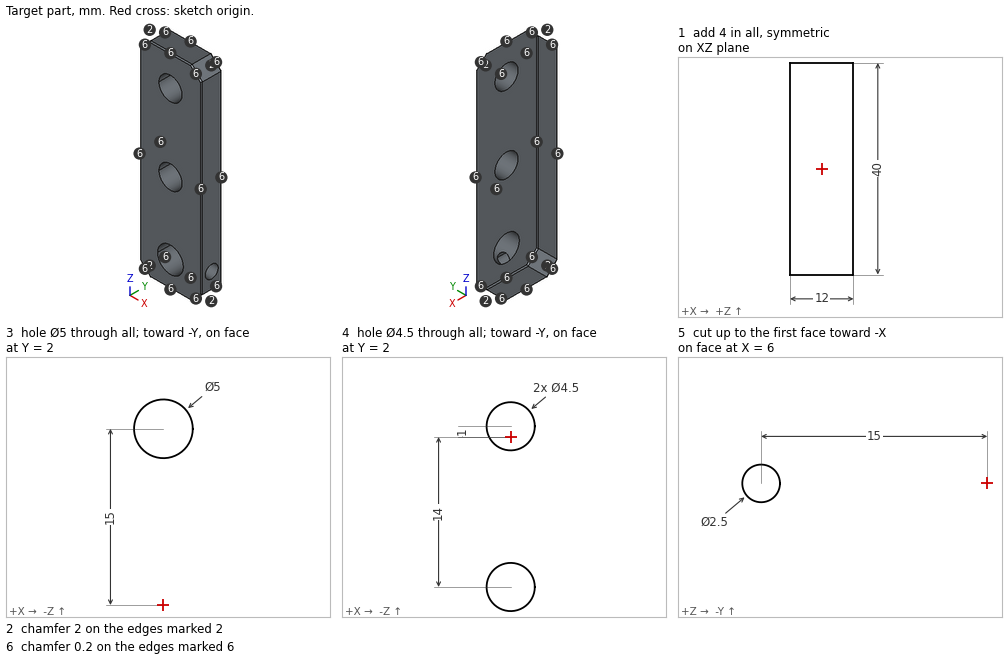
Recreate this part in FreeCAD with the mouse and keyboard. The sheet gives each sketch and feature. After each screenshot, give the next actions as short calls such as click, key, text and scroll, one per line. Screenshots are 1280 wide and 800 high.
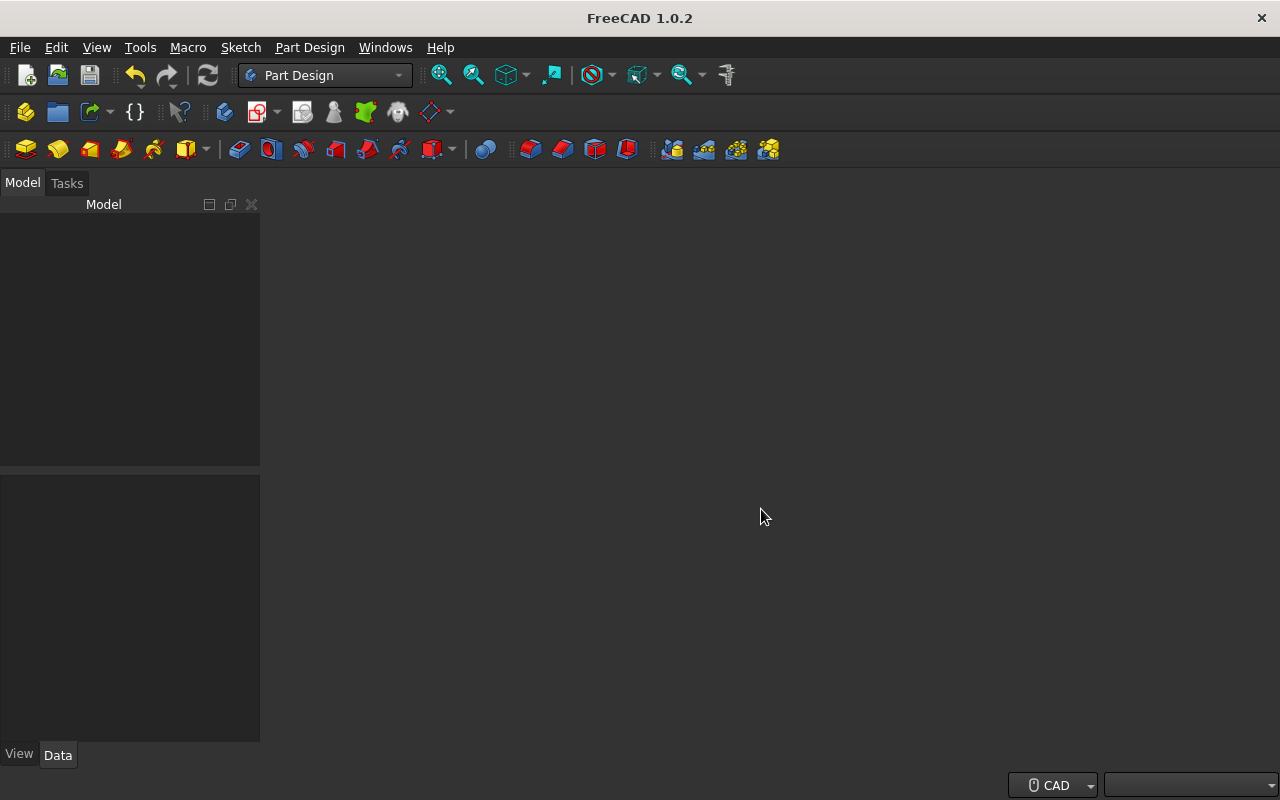
click(26, 76)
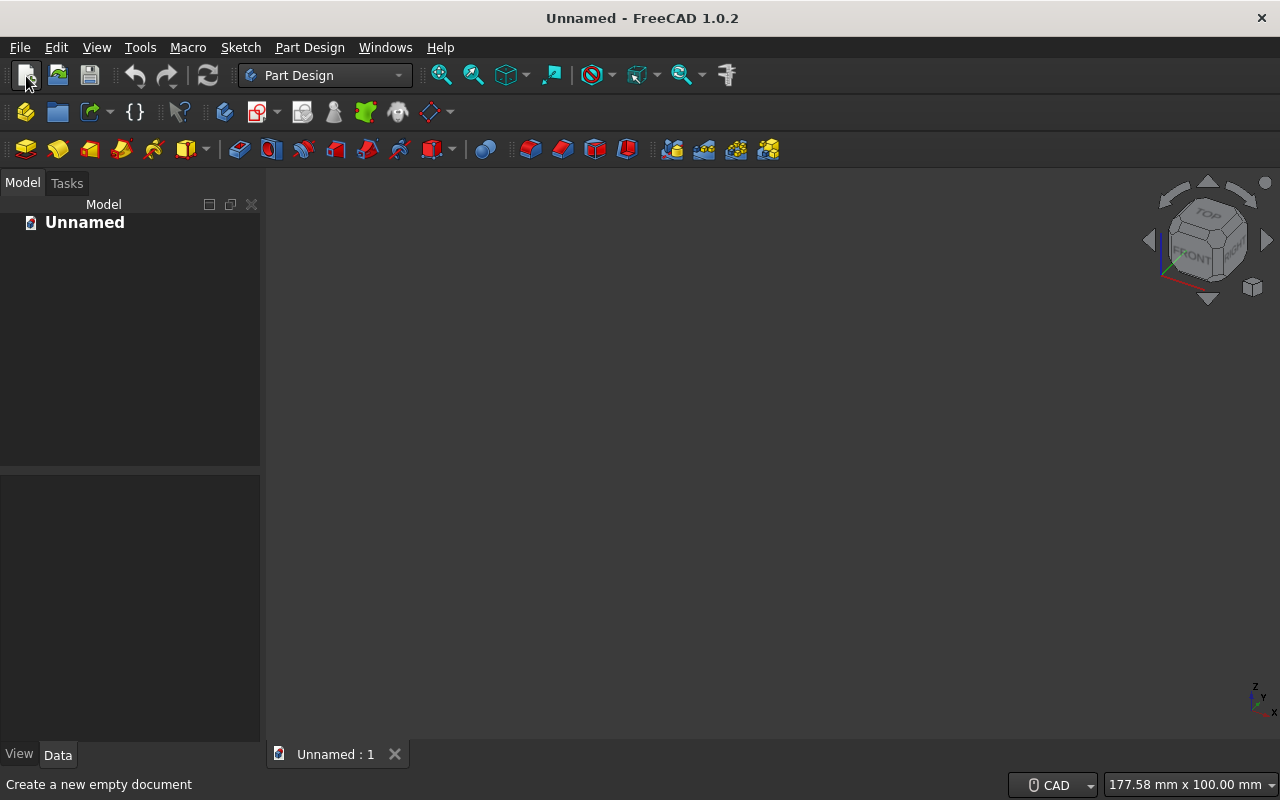
click(258, 112)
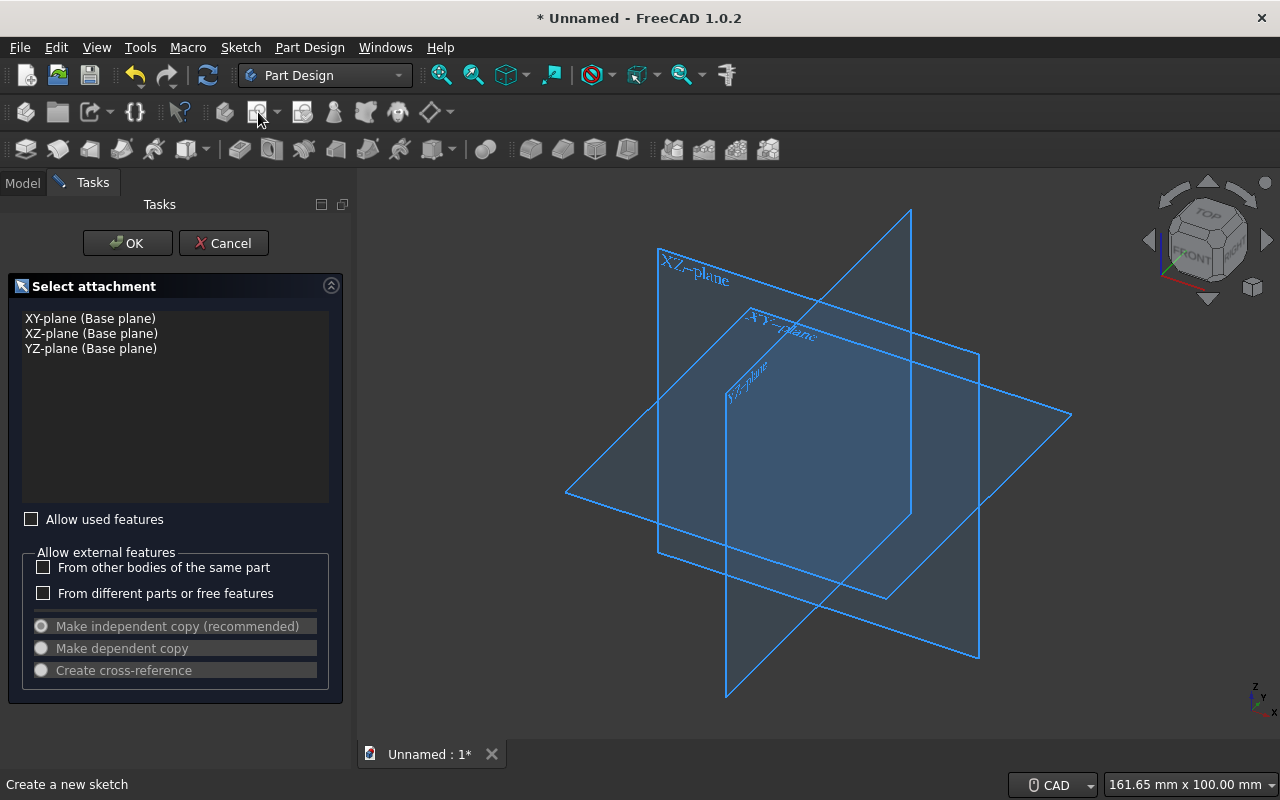
click(82, 334)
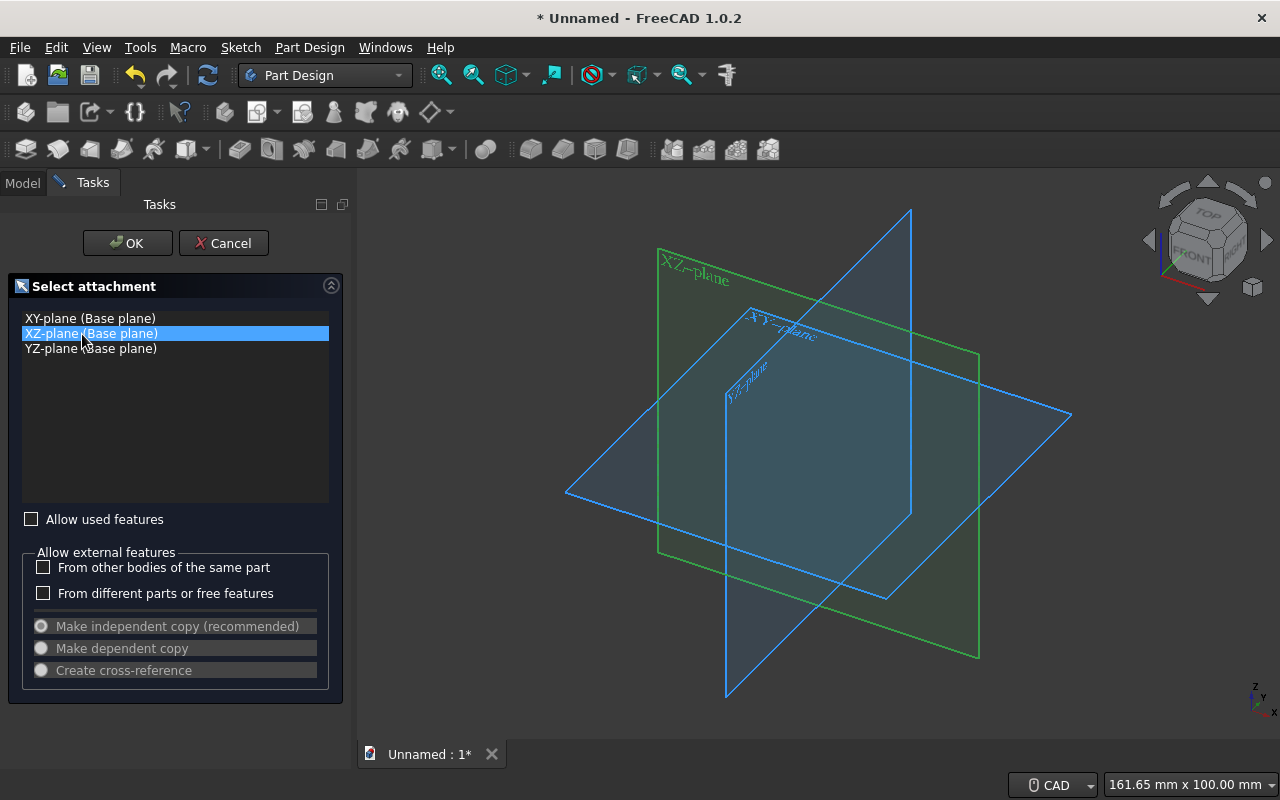
click(128, 243)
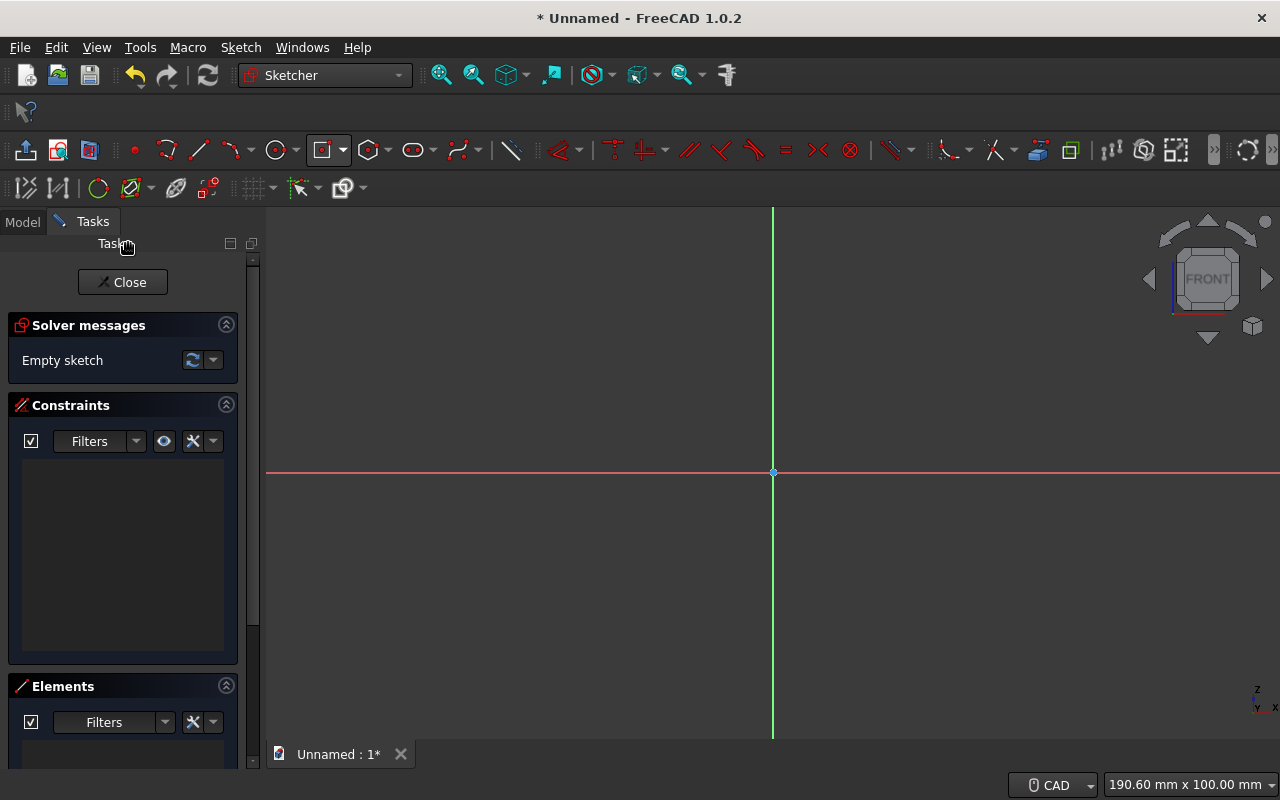
scroll(912, 473, up, 2)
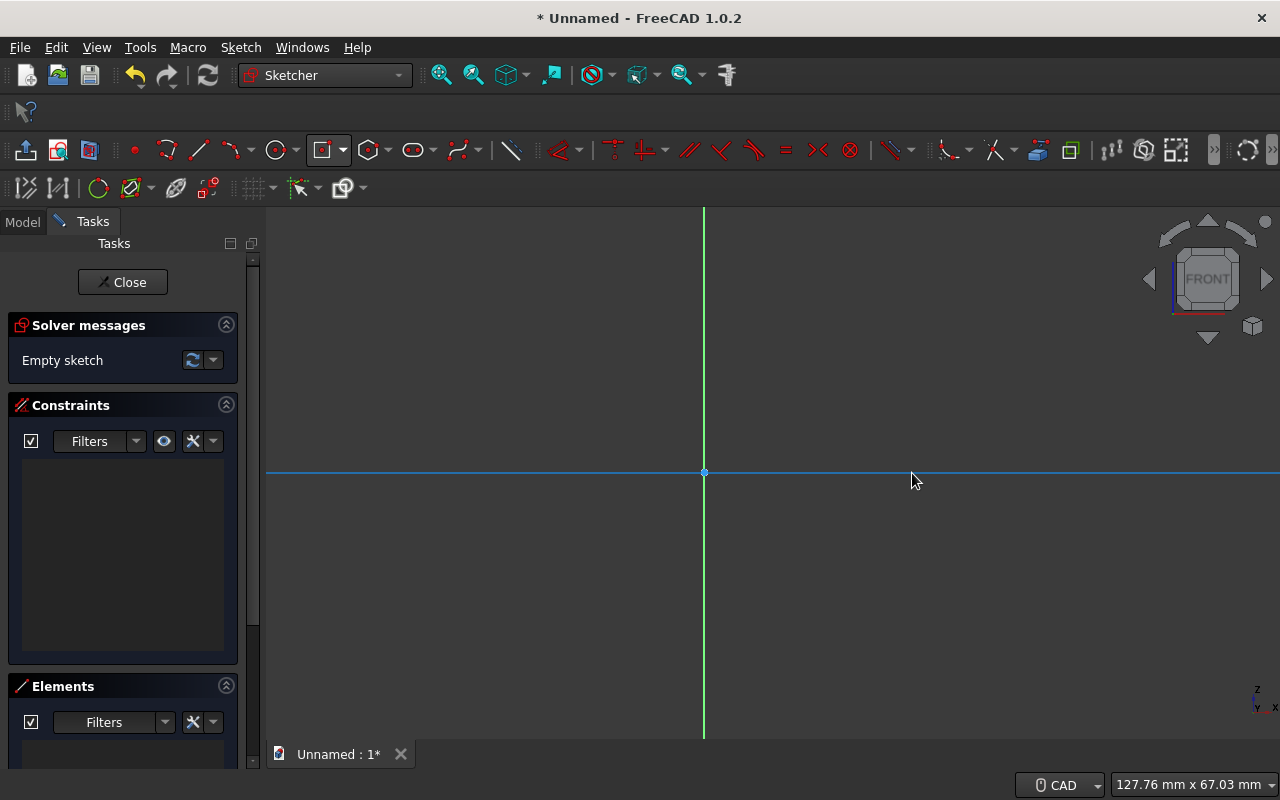
click(322, 150)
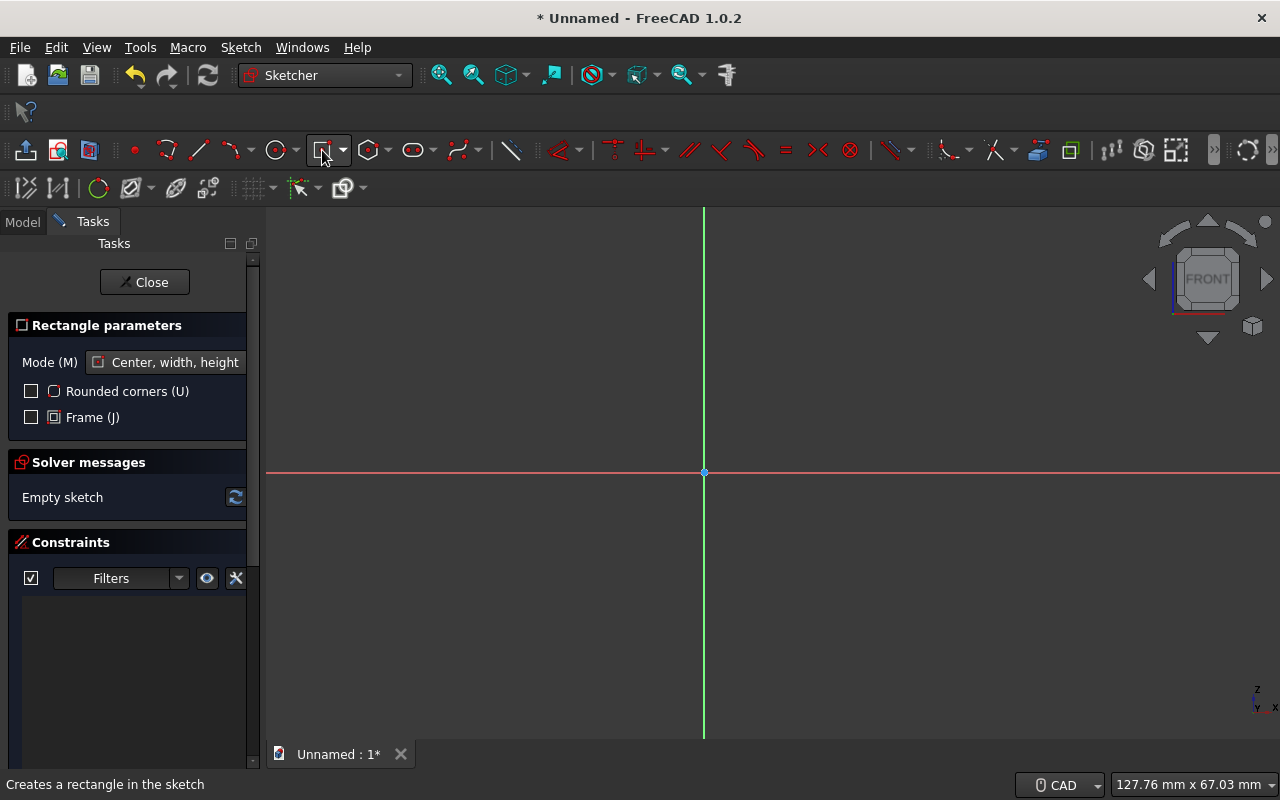
click(704, 473)
click(752, 314)
key(Escape)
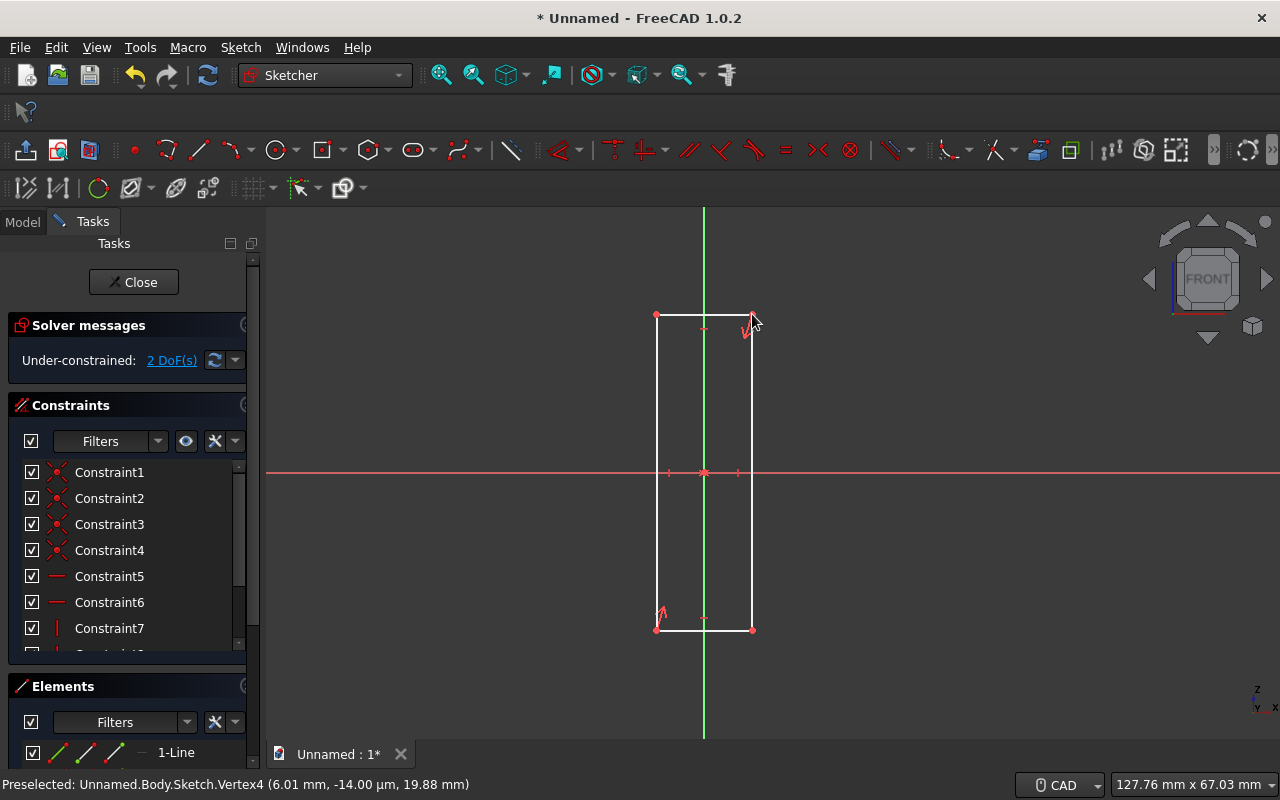
click(558, 150)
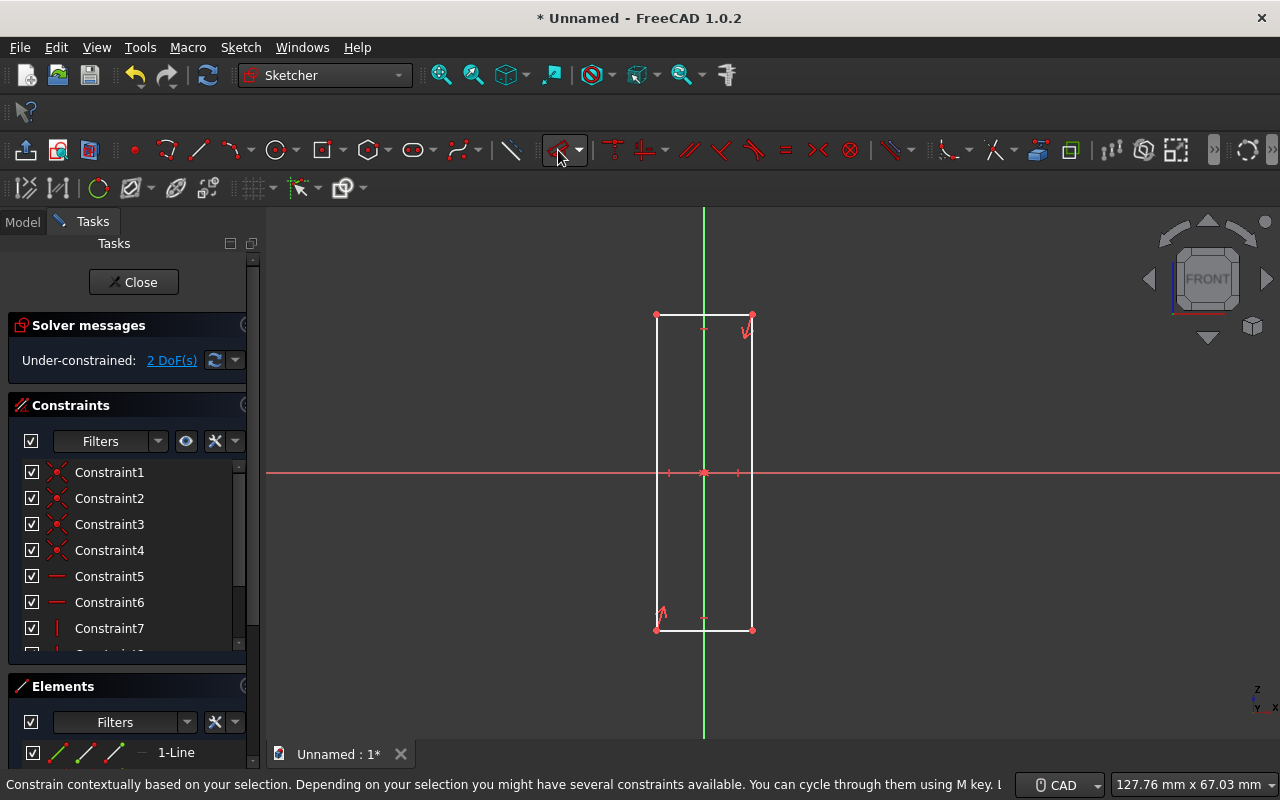
click(685, 631)
click(682, 665)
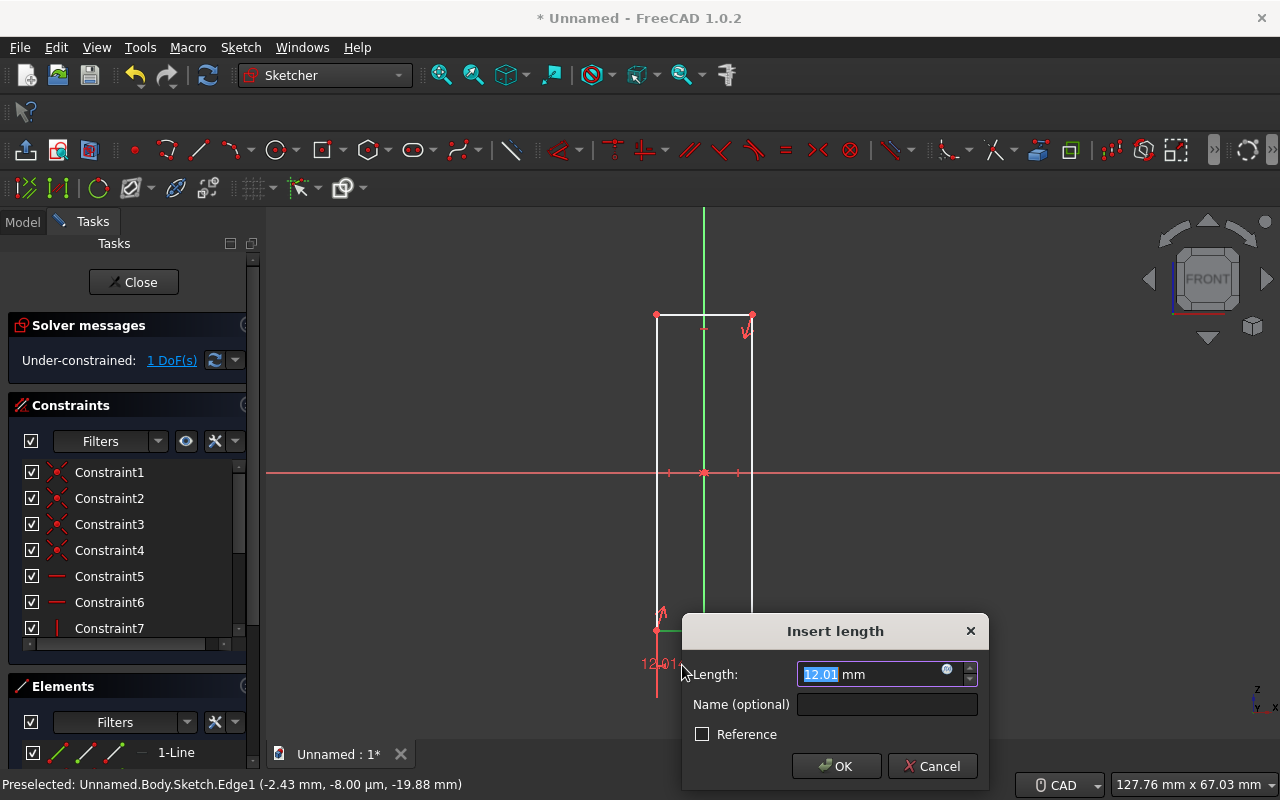
text(12)
key(Return)